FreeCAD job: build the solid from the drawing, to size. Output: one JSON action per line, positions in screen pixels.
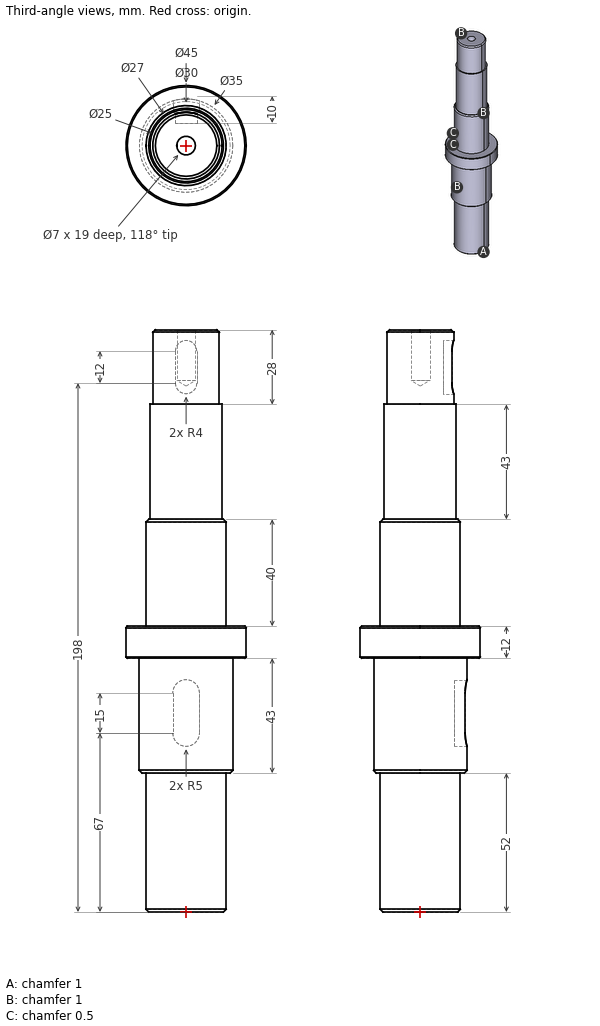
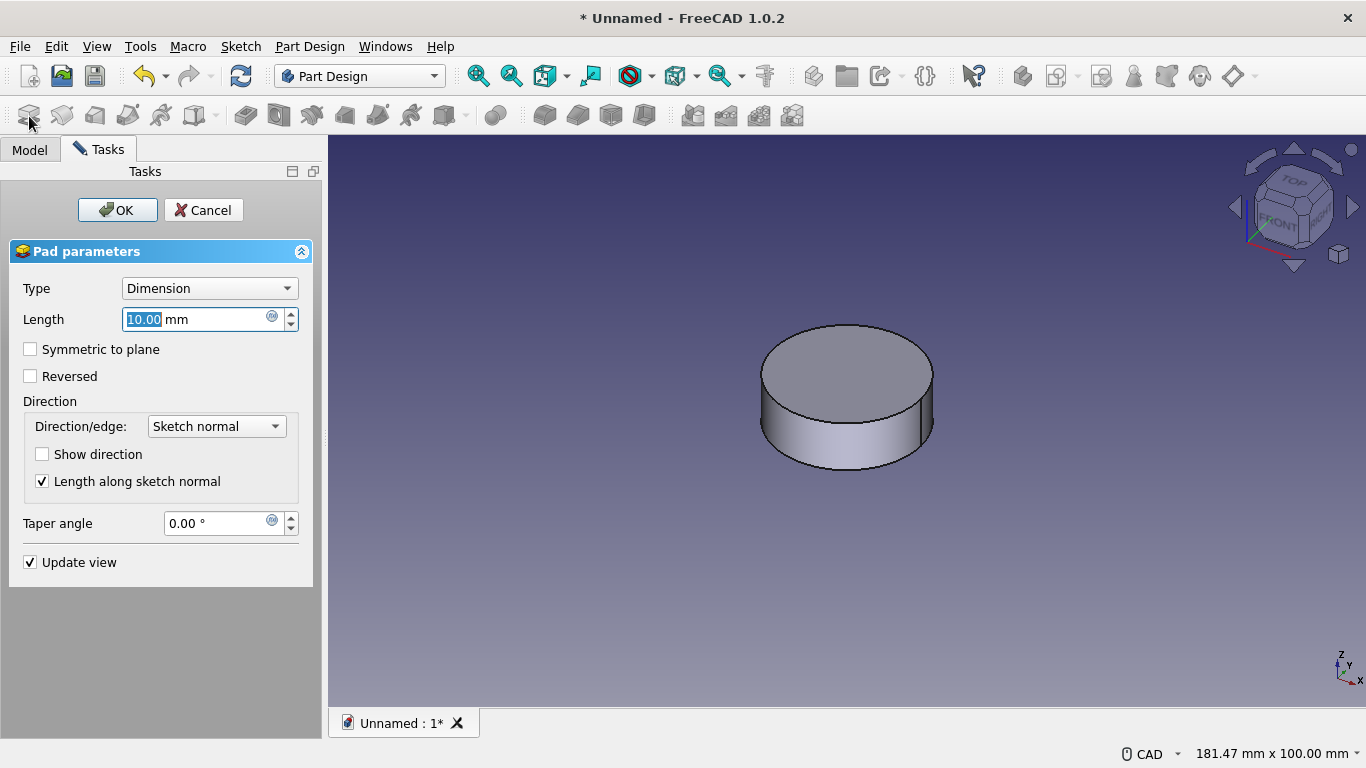
{"action": "type", "text": "52"}
{"action": "key", "text": "Tab"}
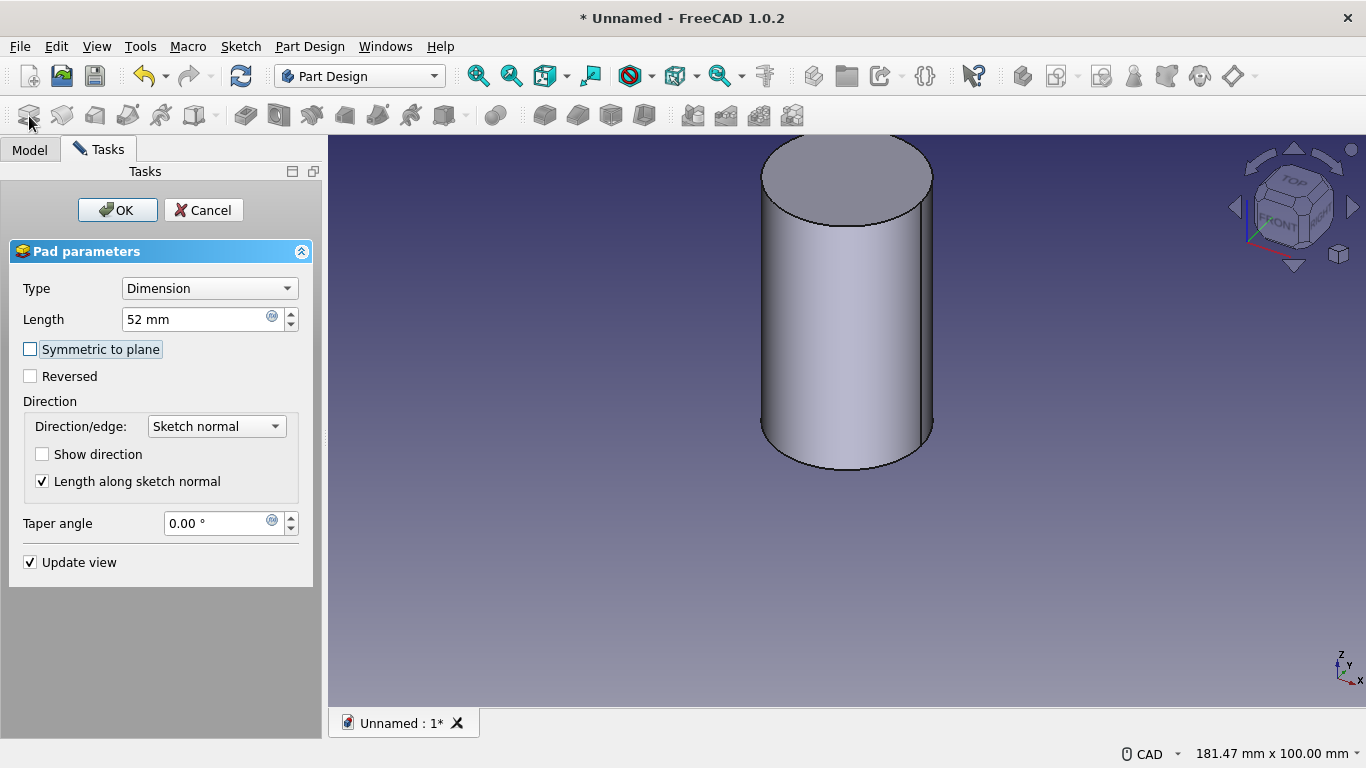
{"action": "left_click", "coordinate": [118, 210]}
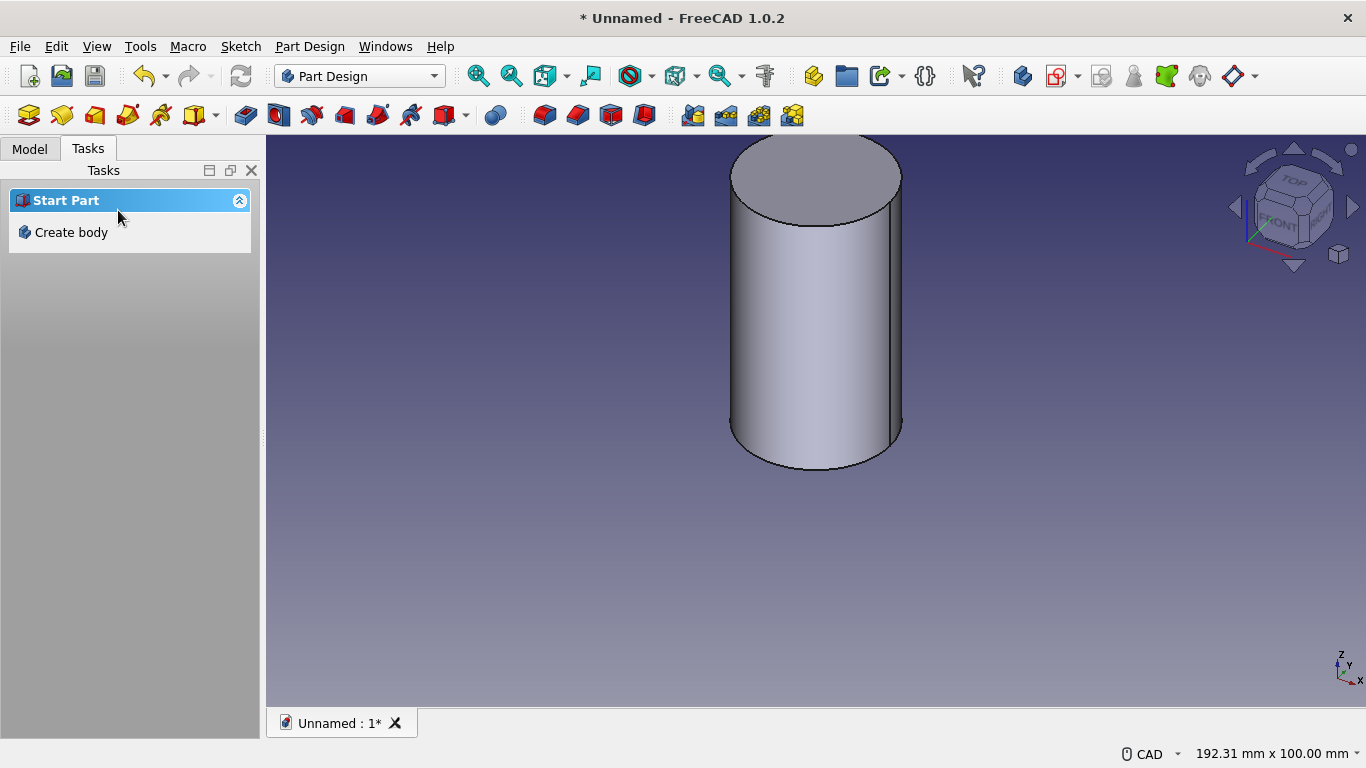
{"action": "left_click", "coordinate": [479, 76]}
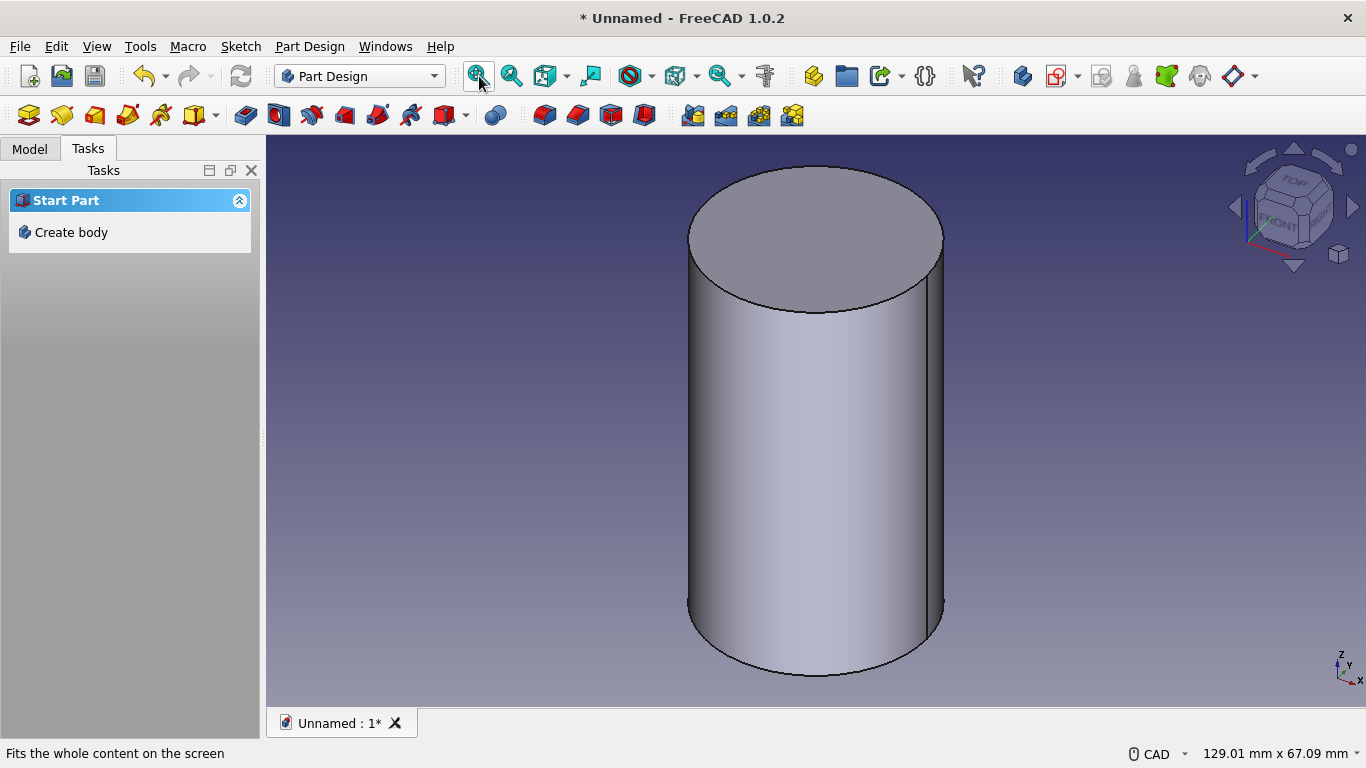
{"action": "left_click", "coordinate": [816, 238]}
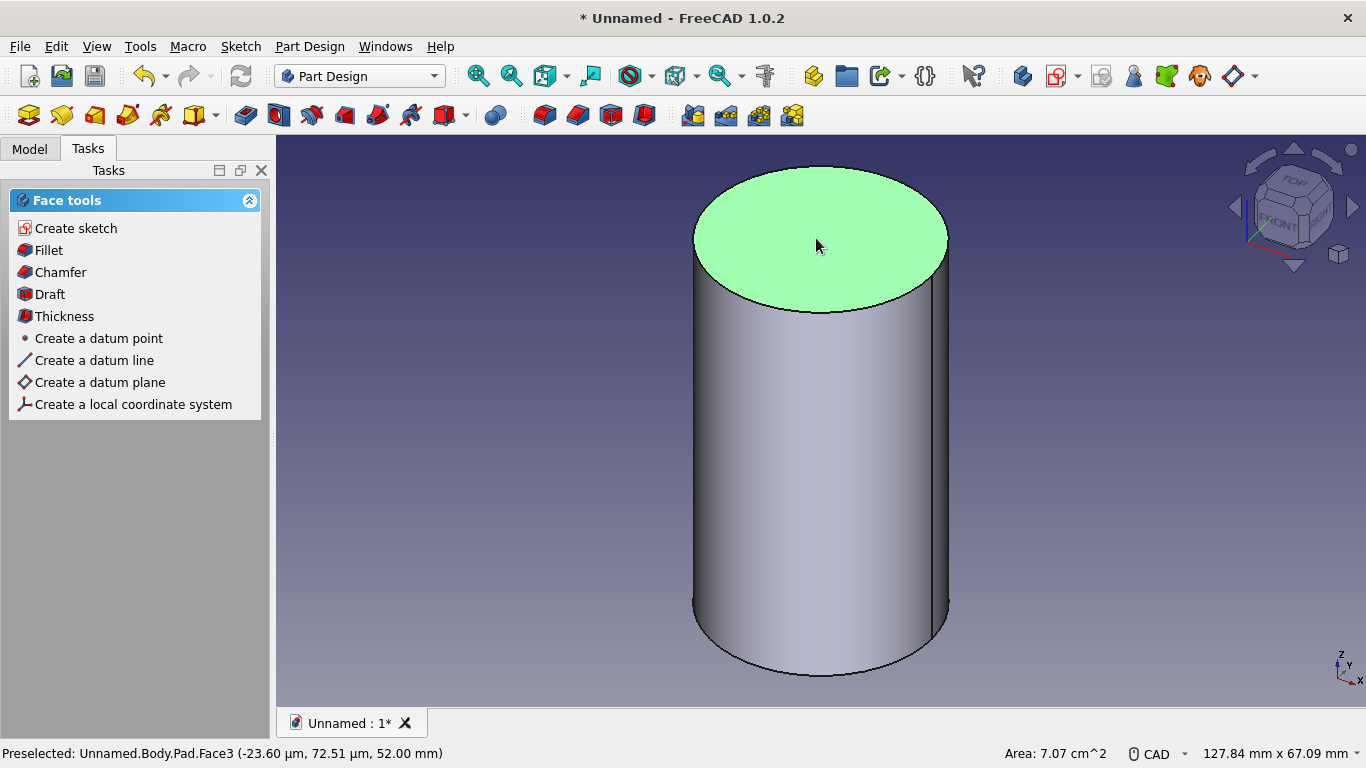
{"action": "left_click", "coordinate": [1056, 76]}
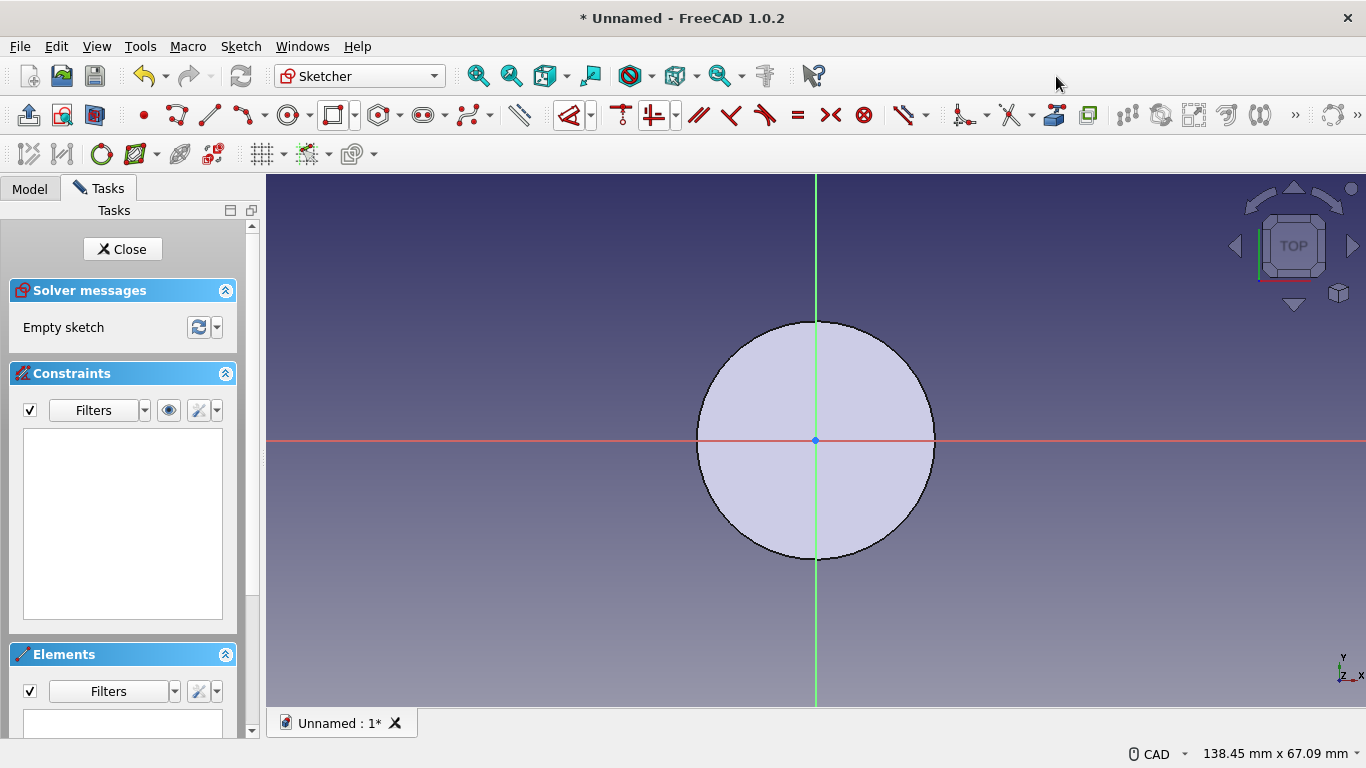
{"action": "key", "text": "g c"}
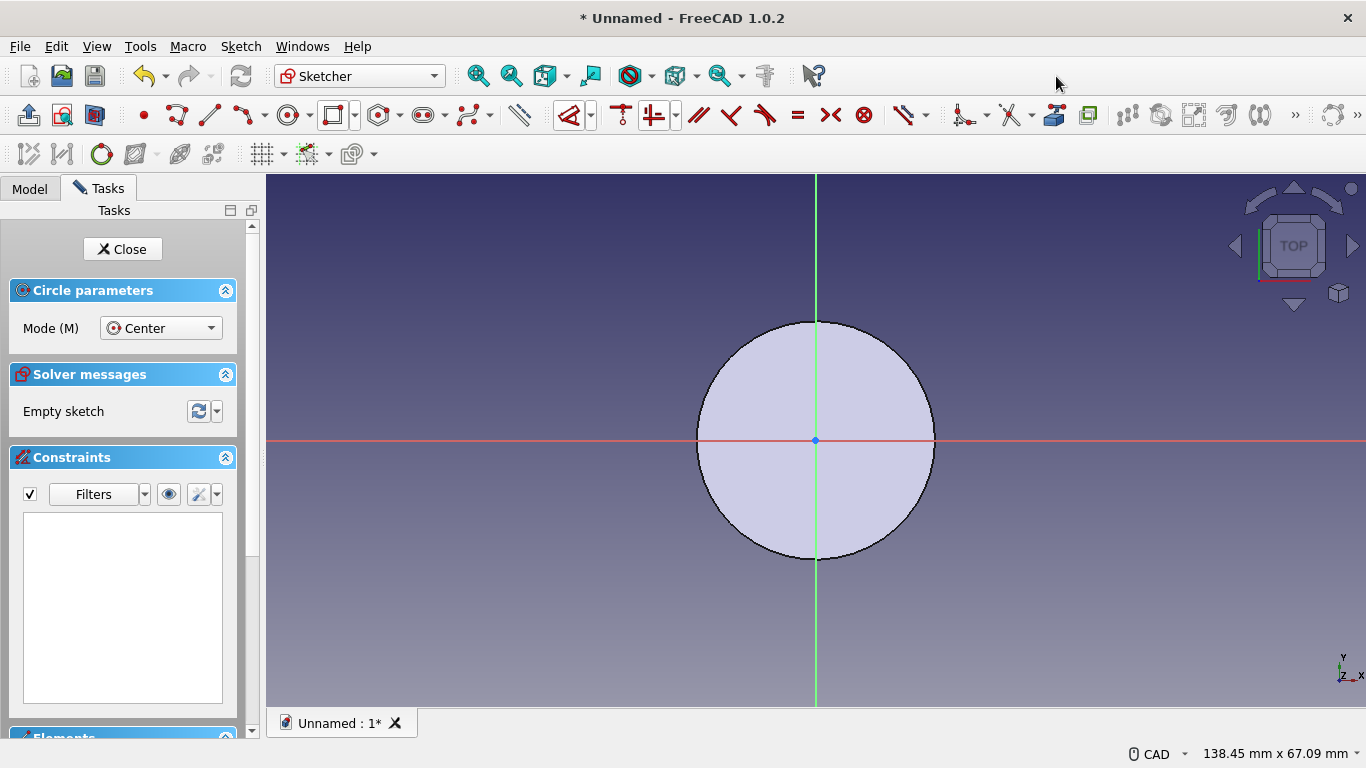
{"action": "left_click", "coordinate": [816, 440]}
{"action": "mouse_move", "coordinate": [914, 342]}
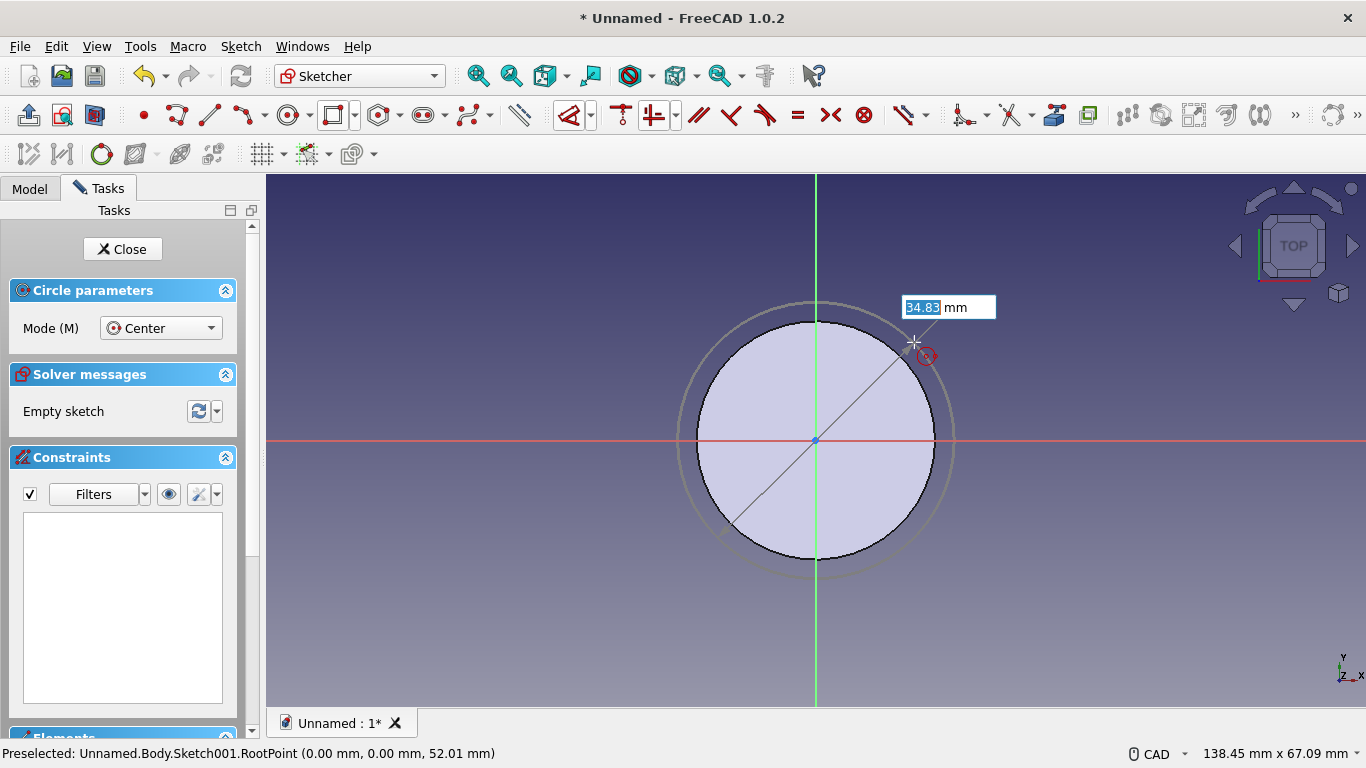
{"action": "type", "text": "35"}
{"action": "key", "text": "Return"}
{"action": "key", "text": "Escape"}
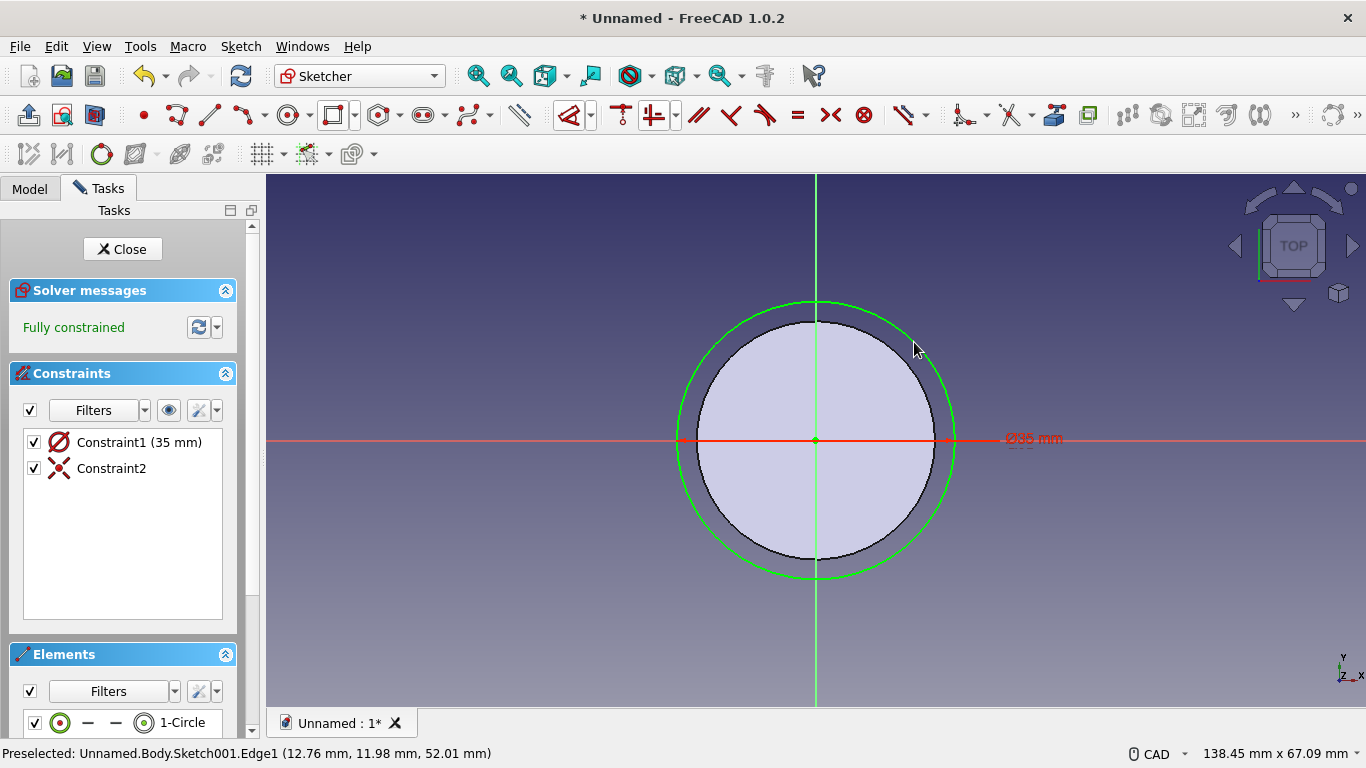
{"action": "left_click", "coordinate": [123, 249]}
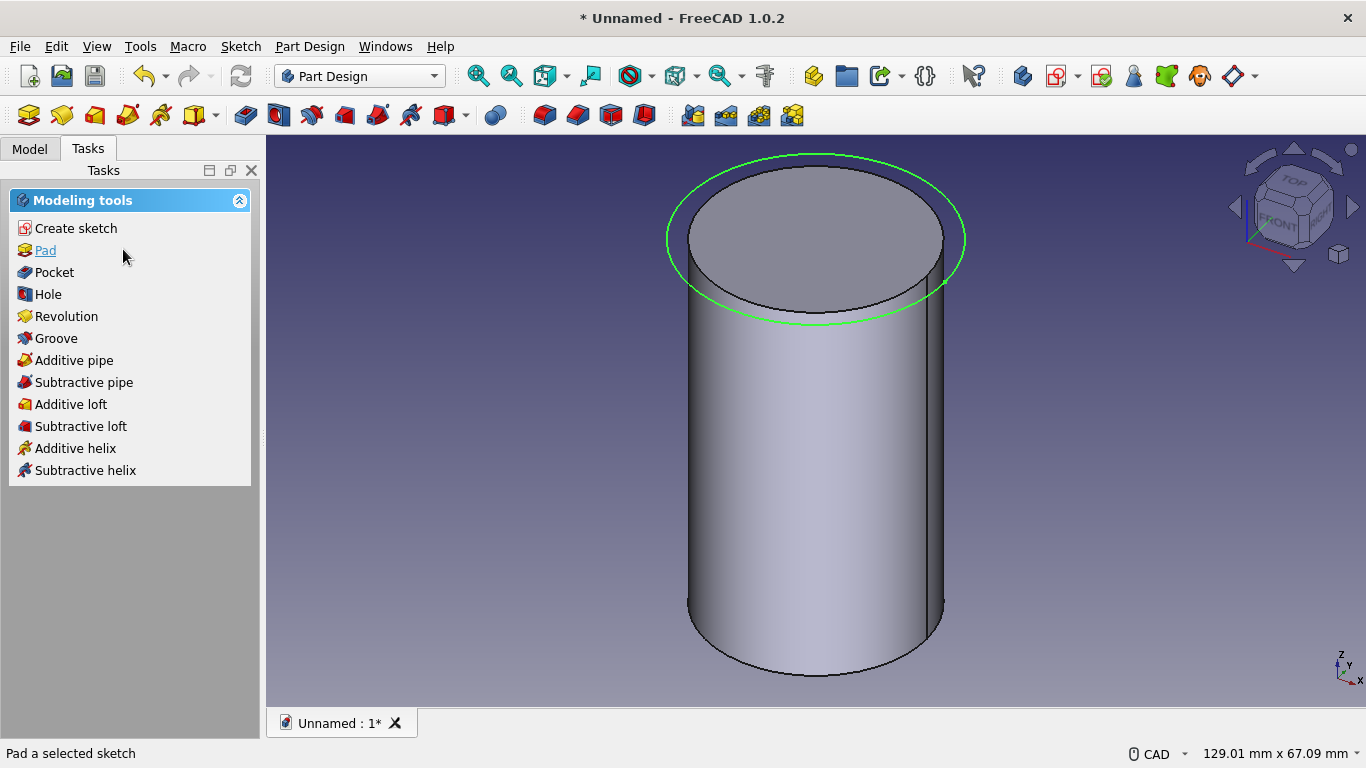
{"action": "left_click", "coordinate": [29, 116]}